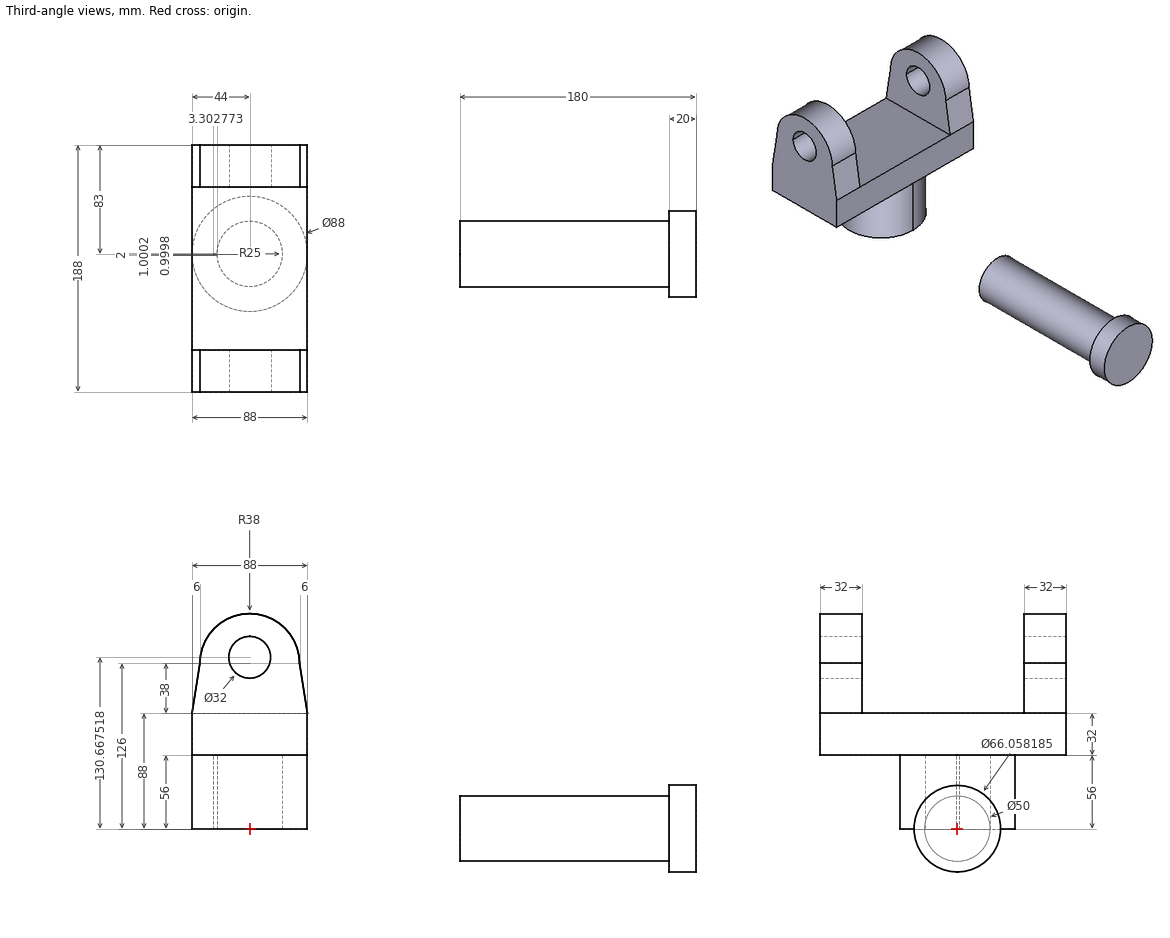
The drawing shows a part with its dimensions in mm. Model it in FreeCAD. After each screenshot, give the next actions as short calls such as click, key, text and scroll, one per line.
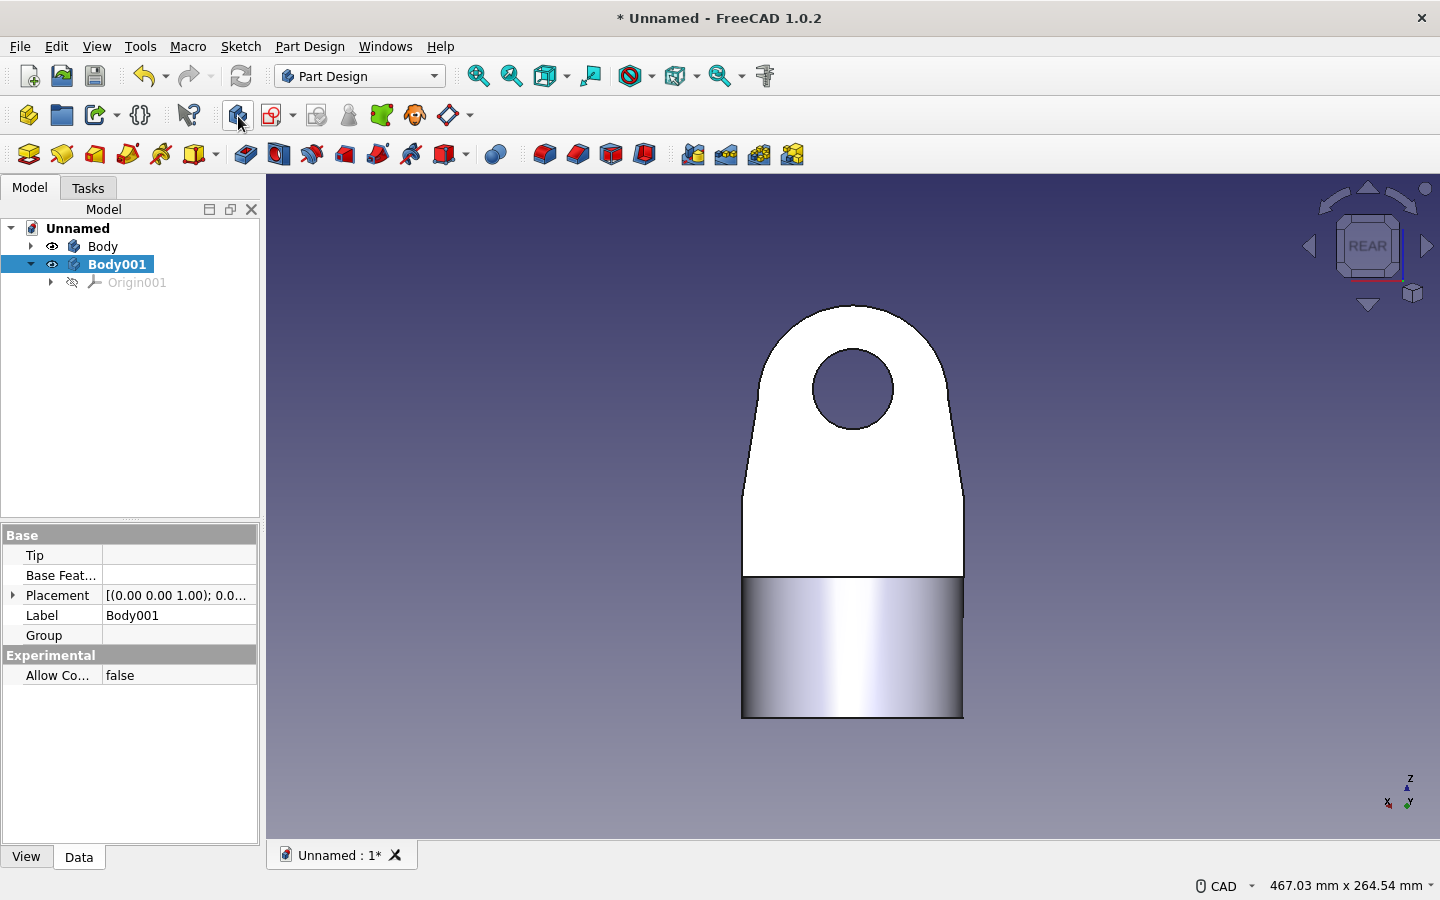
click(51, 282)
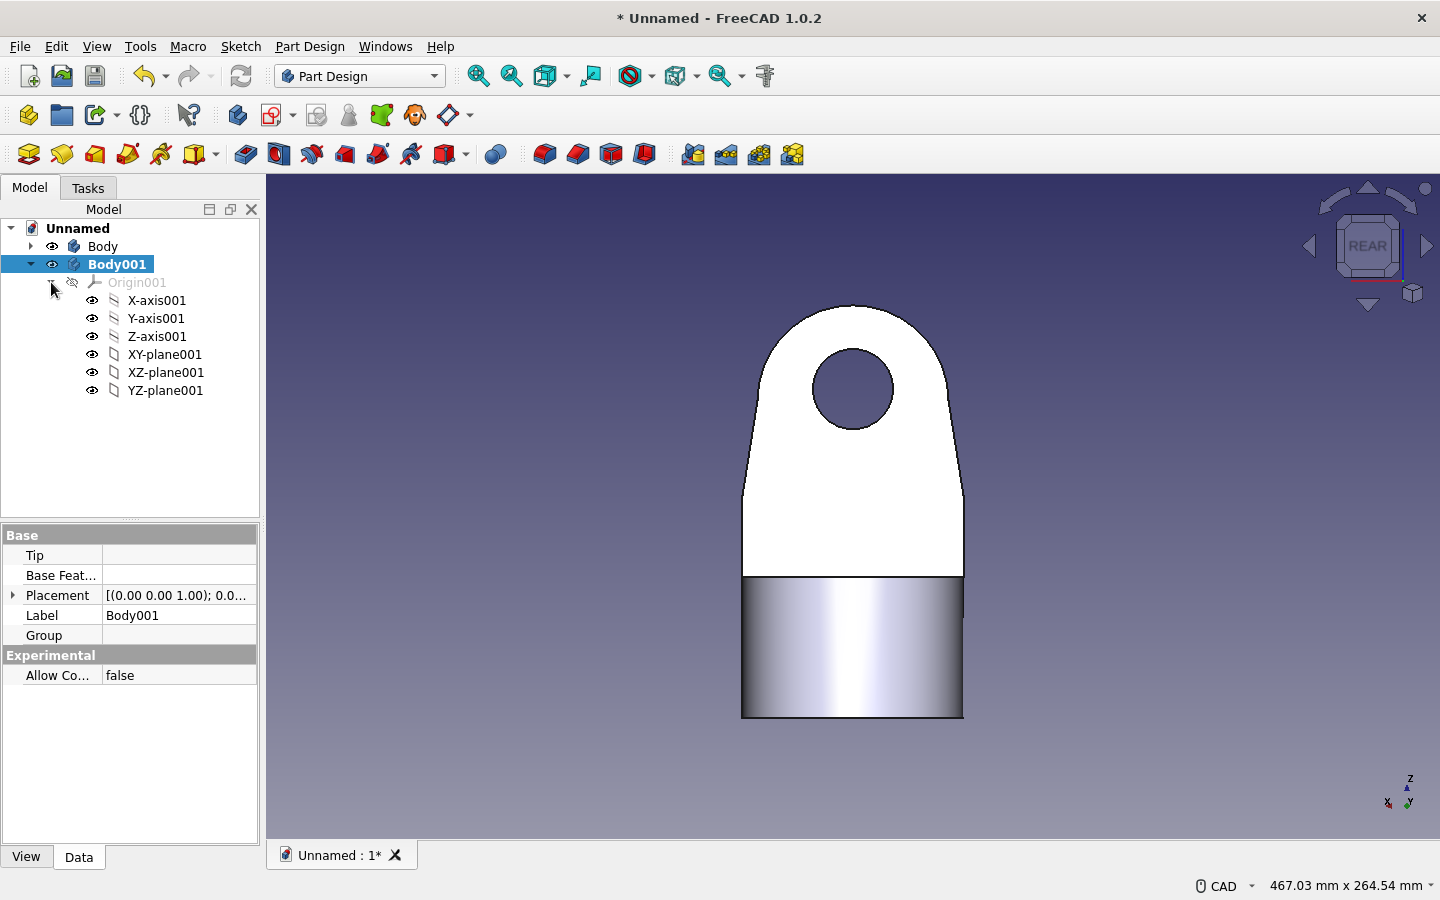
click(137, 390)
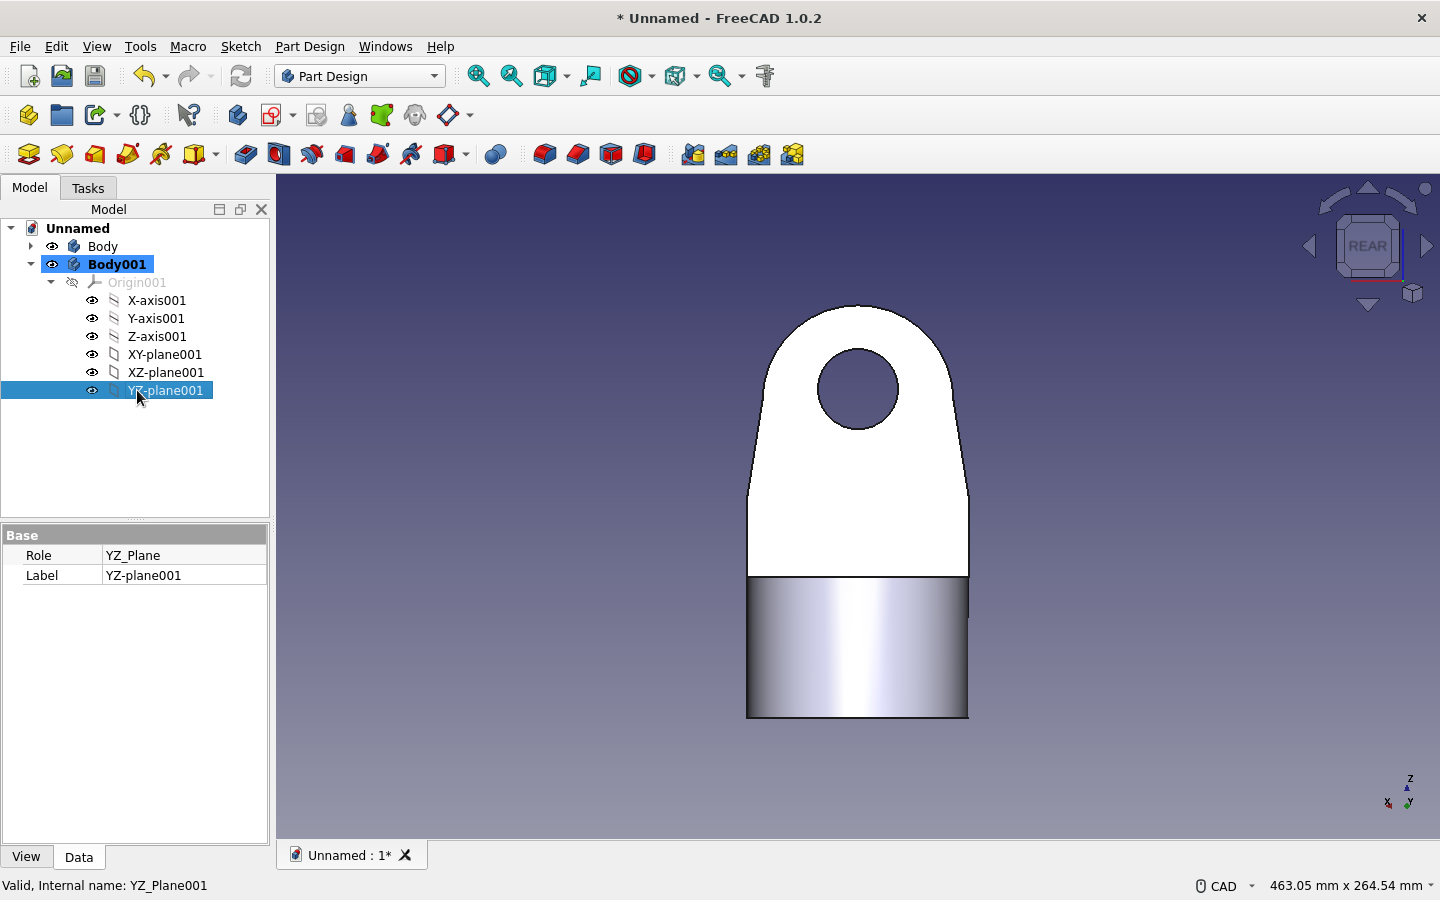
click(448, 116)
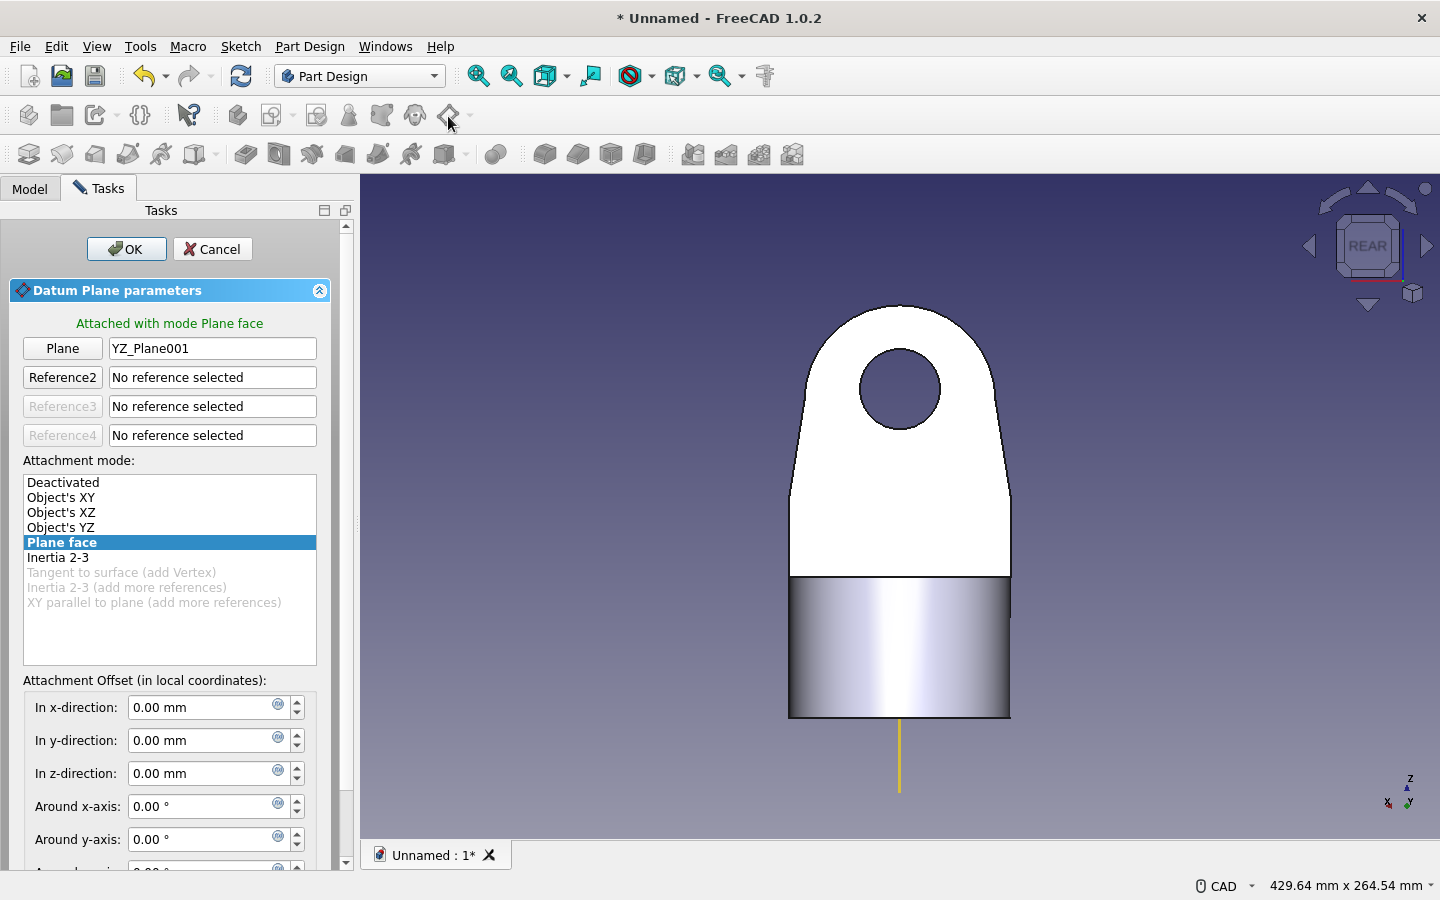
triple_click(210, 774)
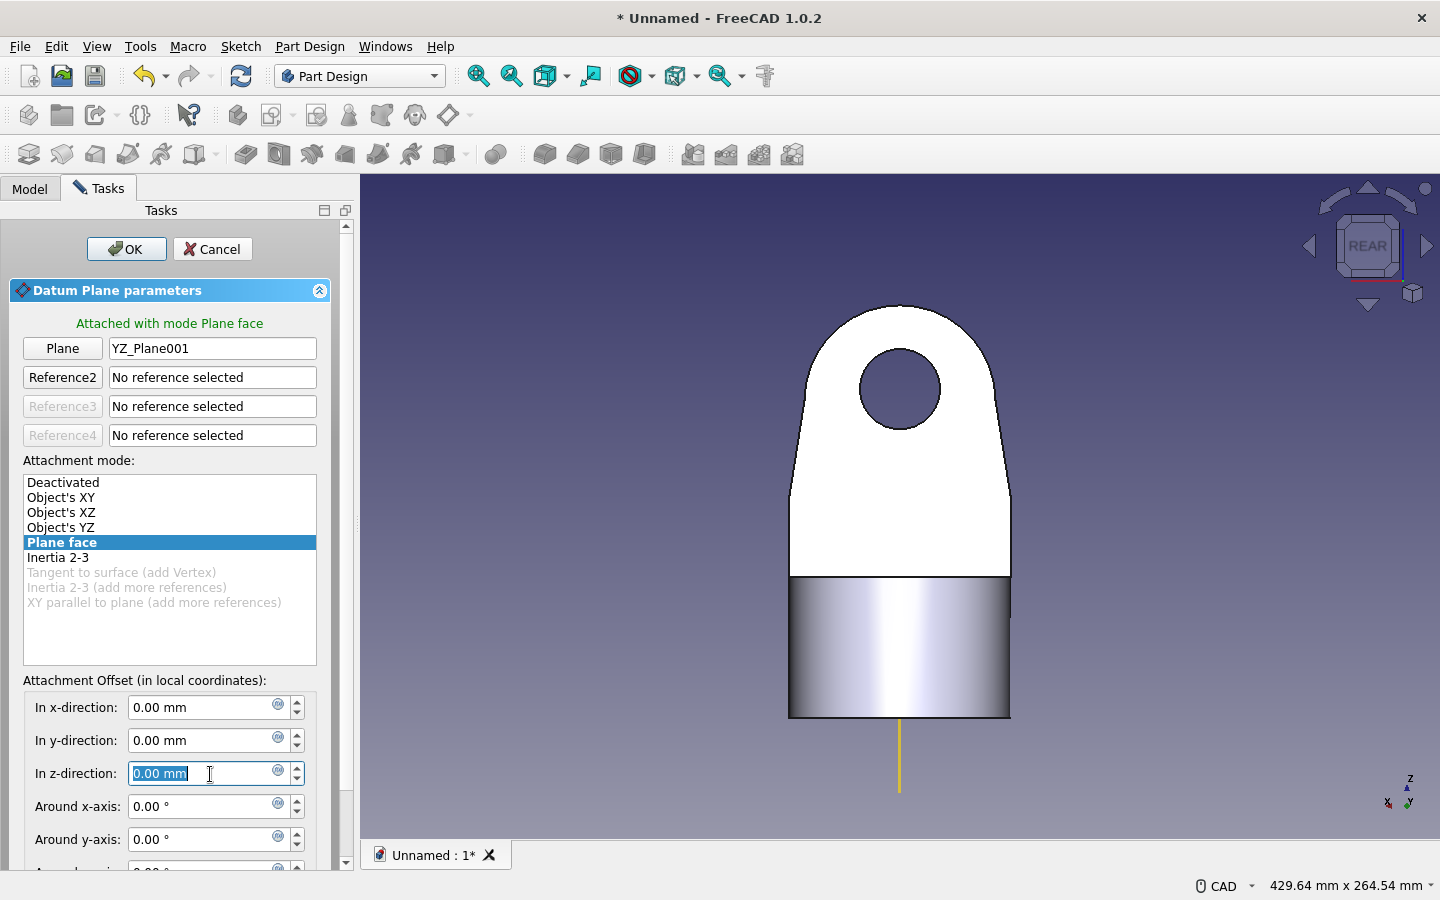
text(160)
key(Tab)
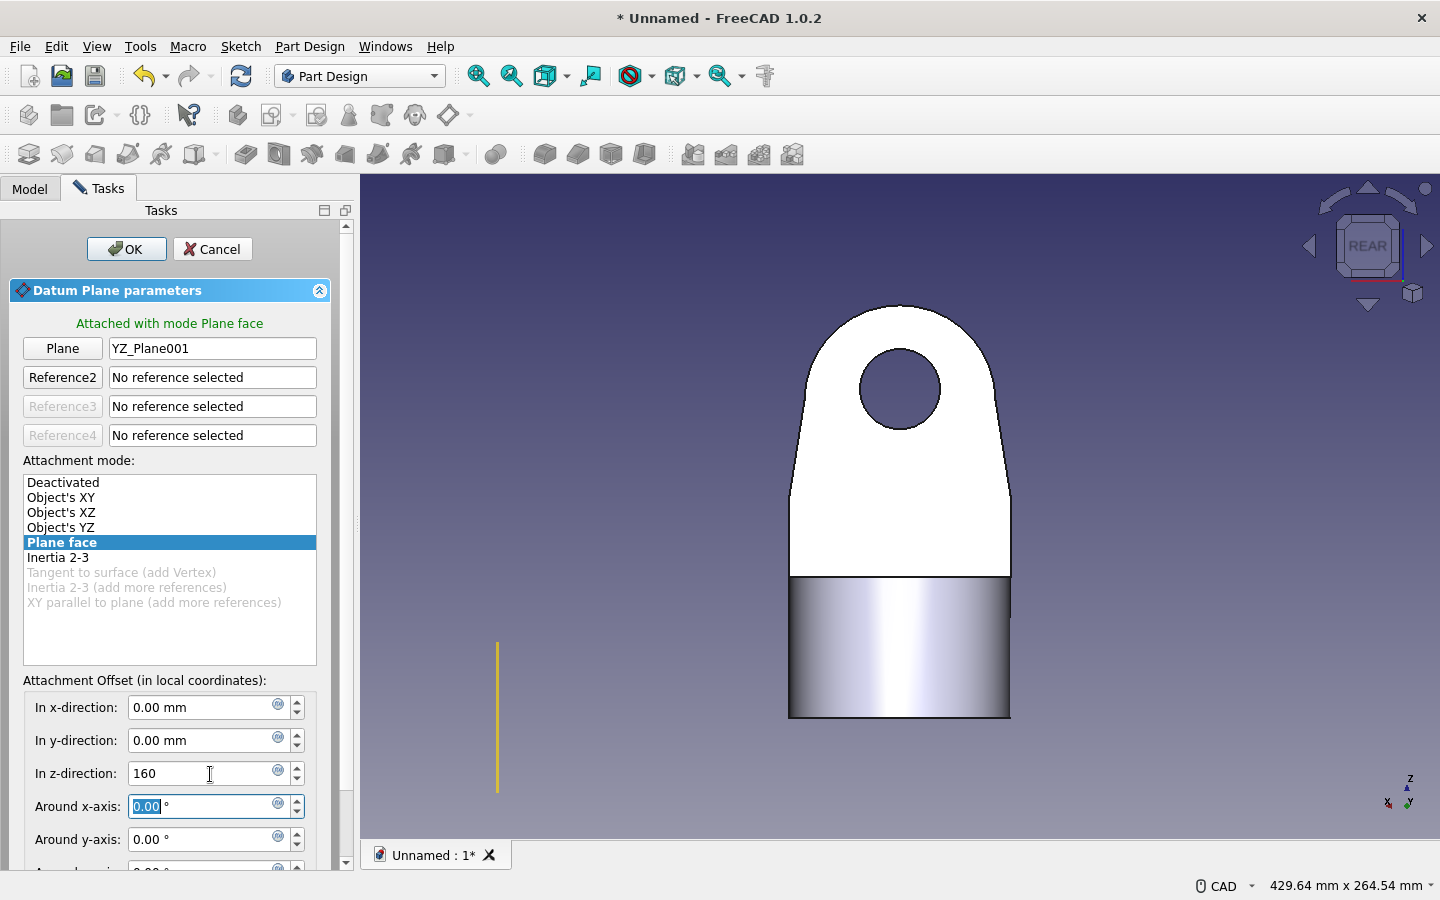
click(127, 249)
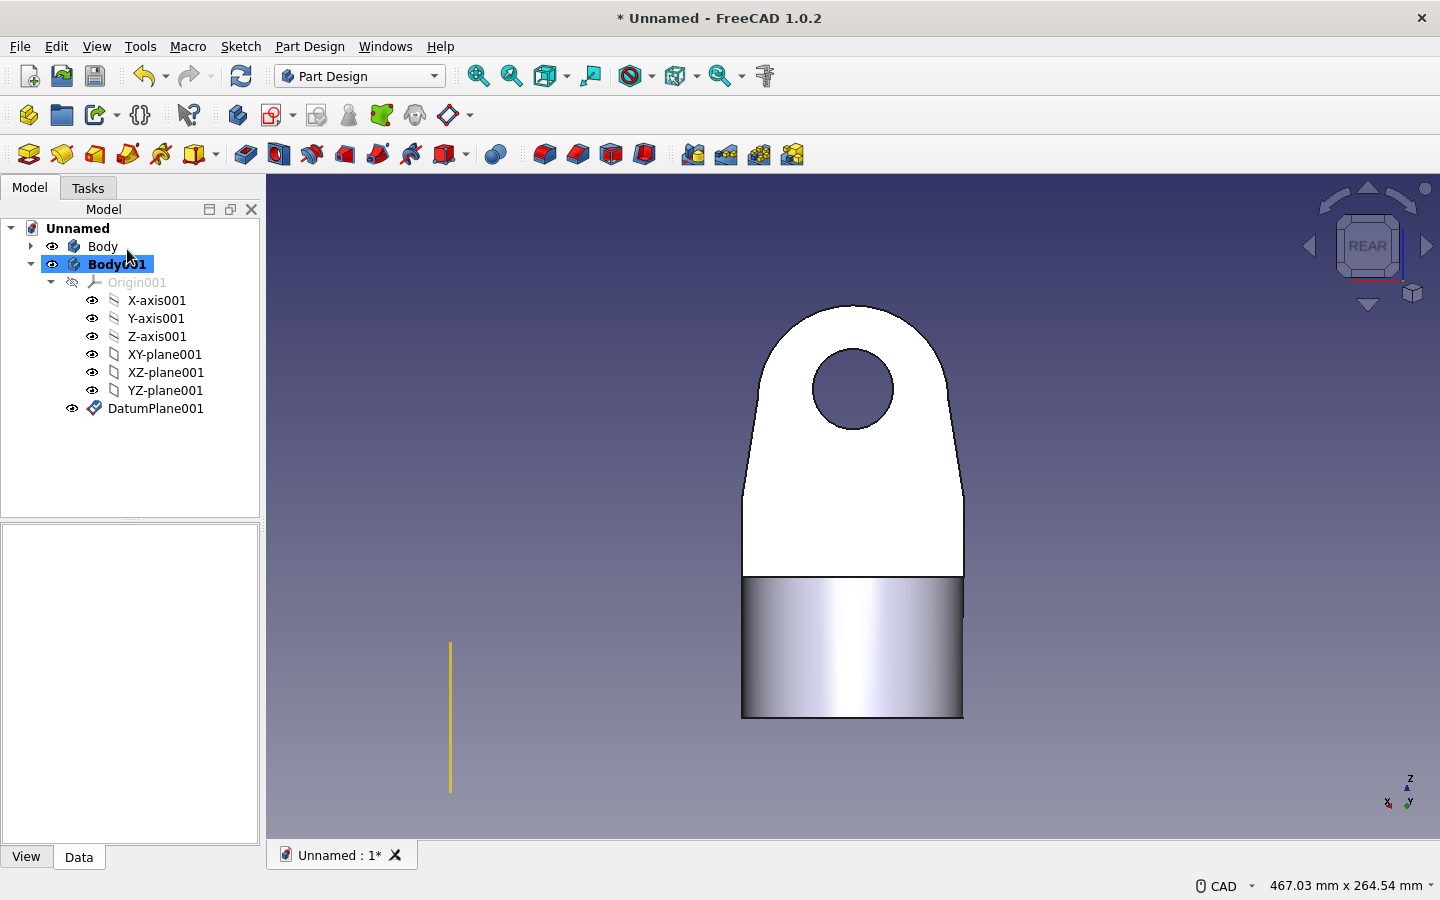
click(117, 408)